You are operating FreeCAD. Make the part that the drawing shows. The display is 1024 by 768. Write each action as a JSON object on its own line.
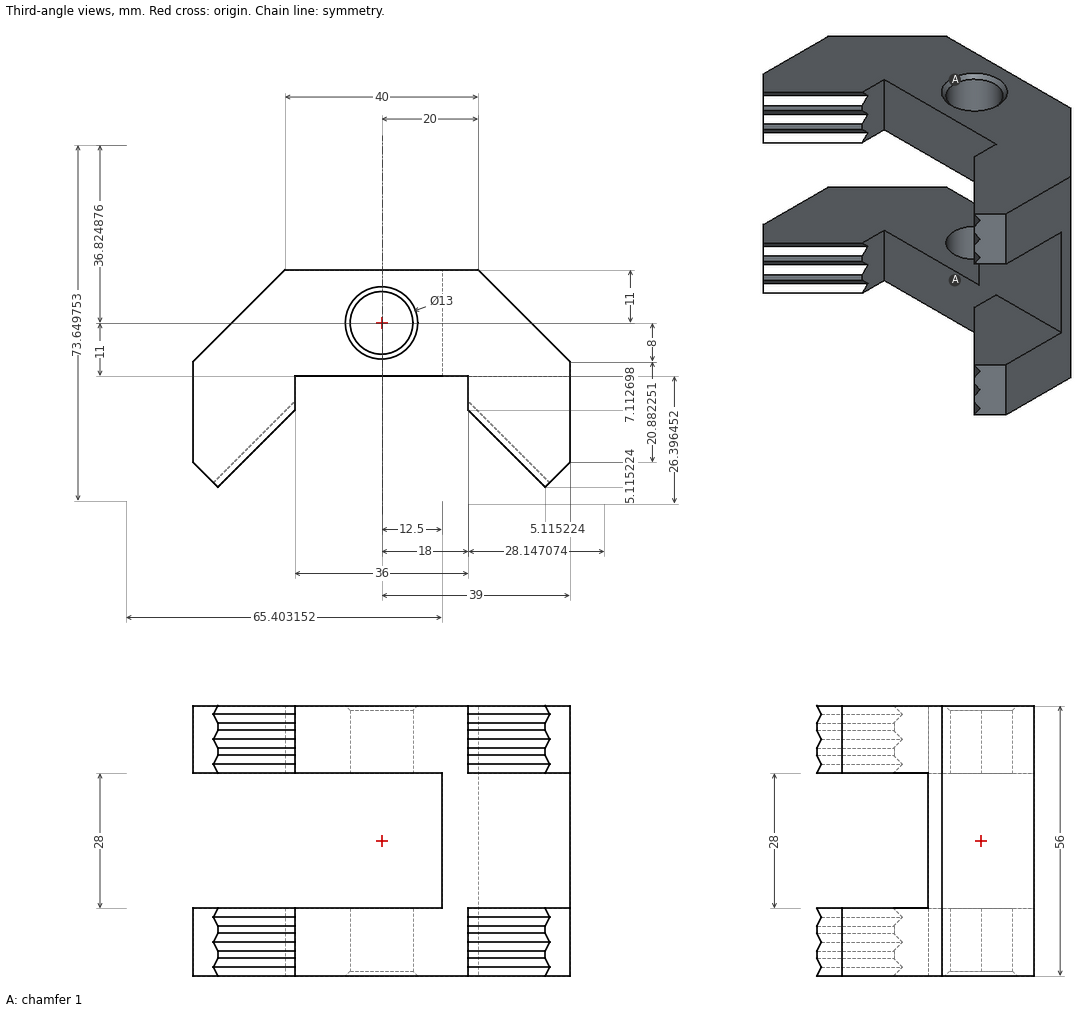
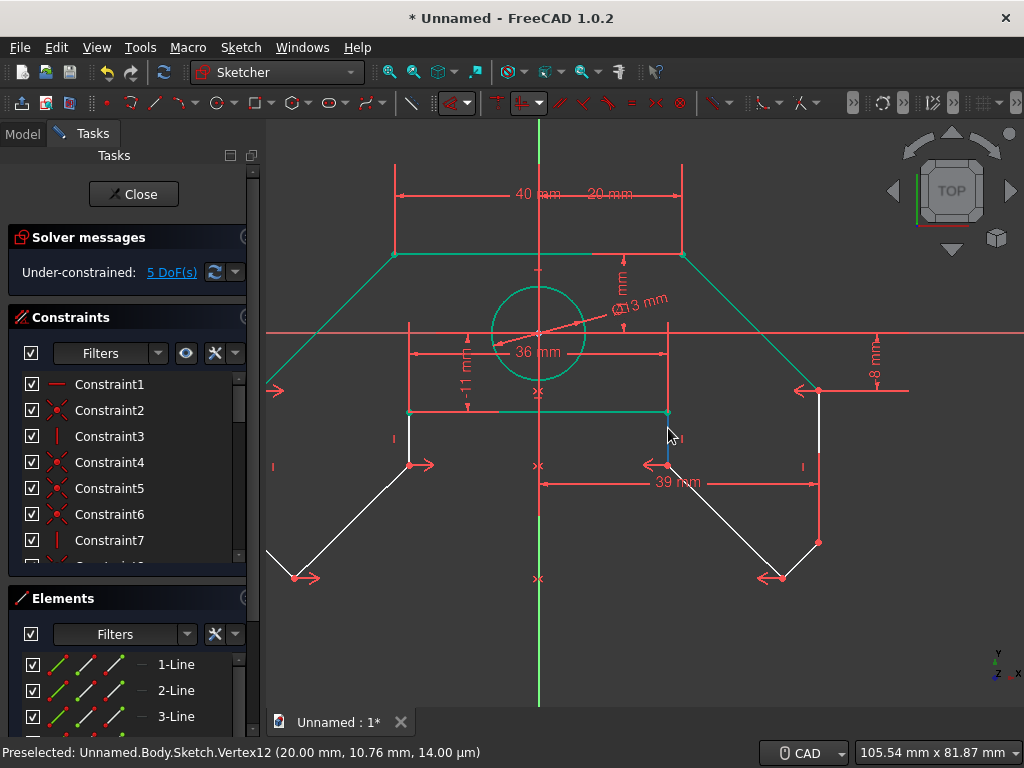
{"action": "left_click", "coordinate": [668, 428]}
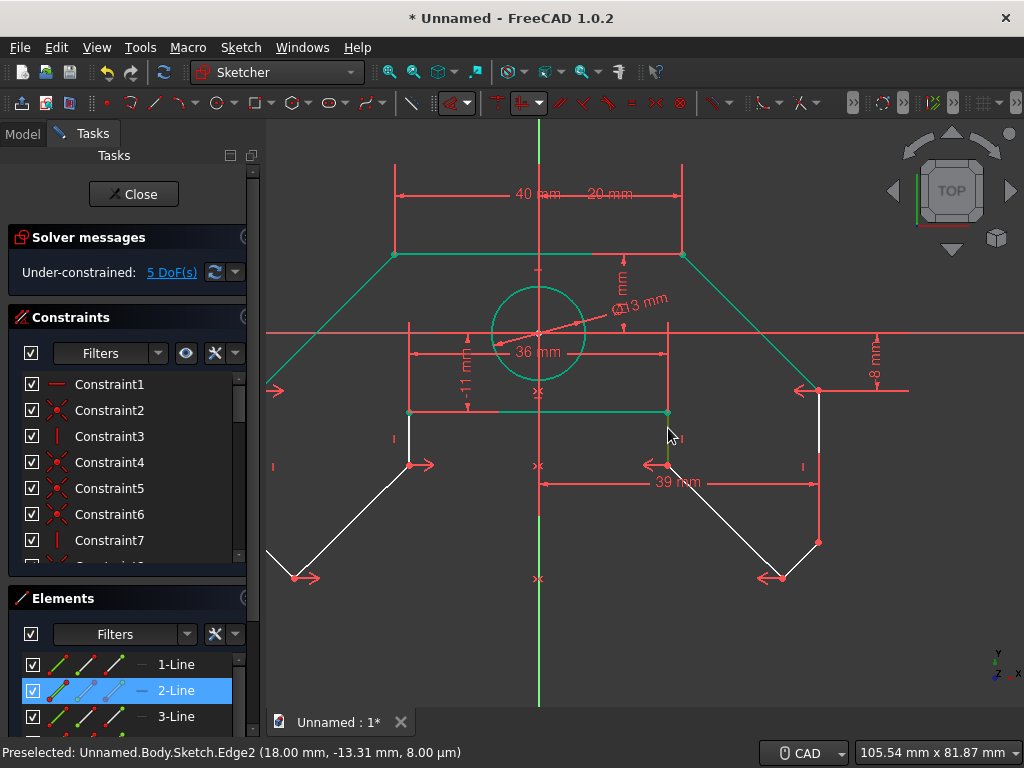
{"action": "key", "text": "i"}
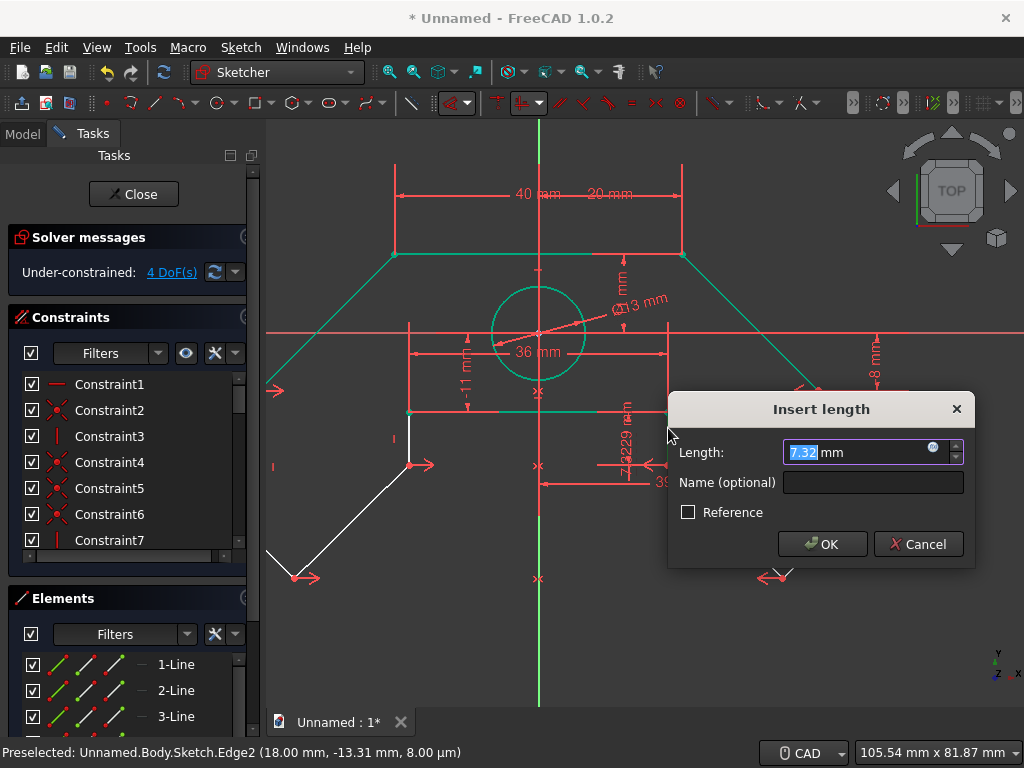
{"action": "type", "text": "7.112698"}
{"action": "key", "text": "Return"}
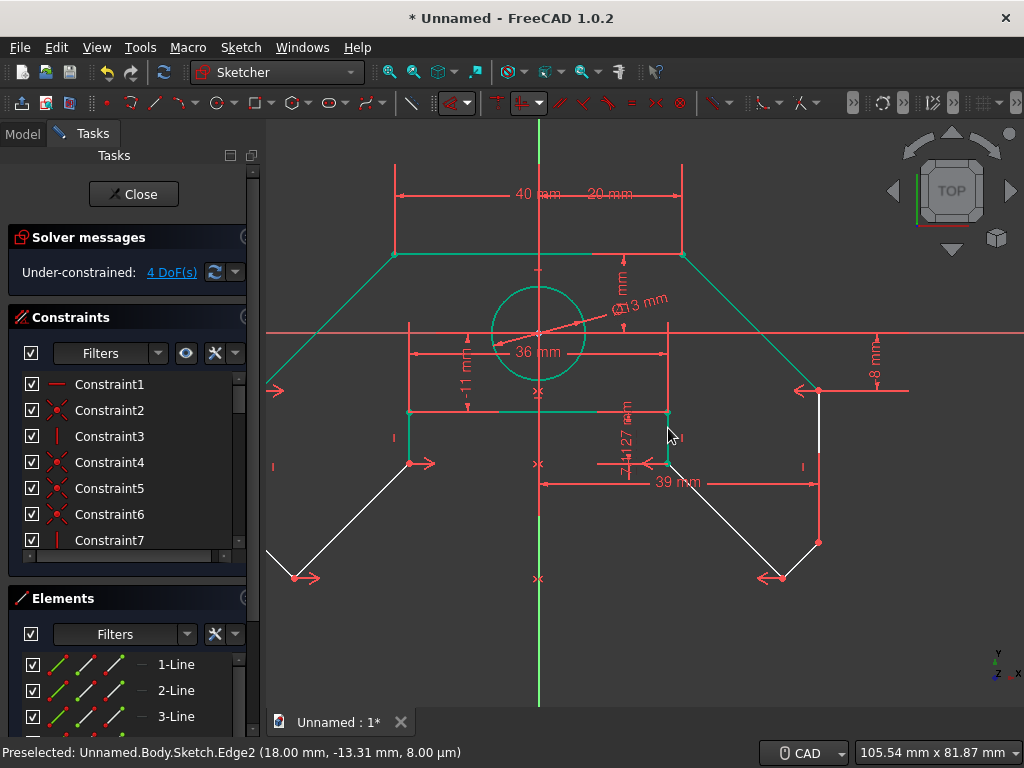
{"action": "left_click", "coordinate": [819, 497]}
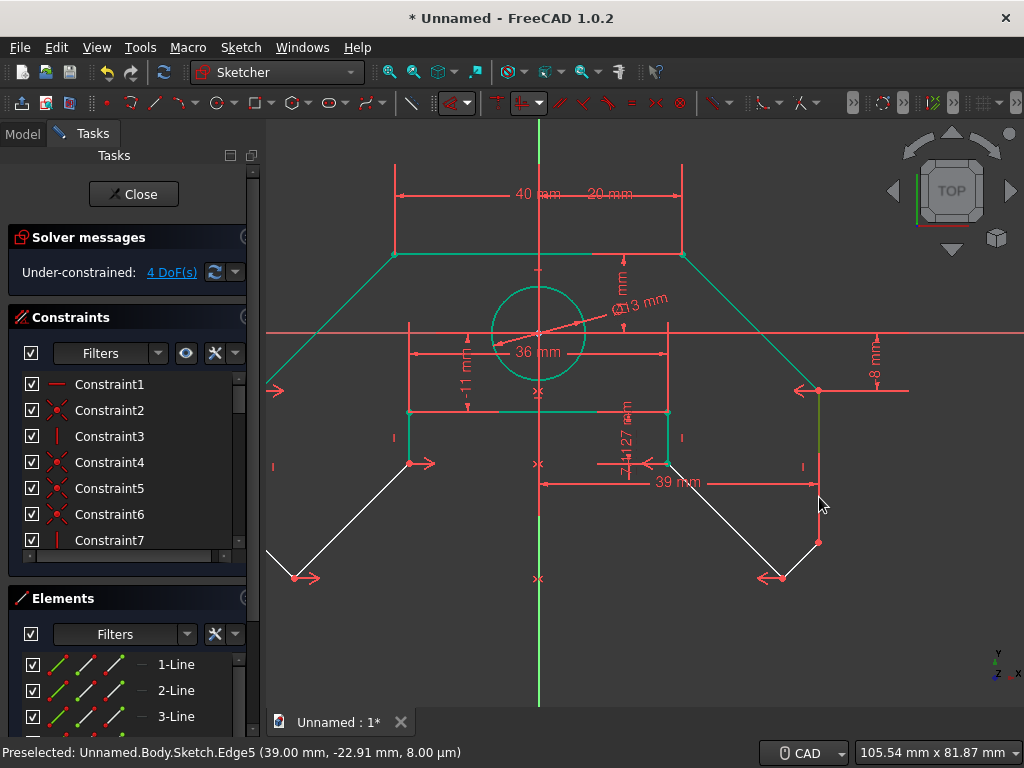
{"action": "key", "text": "i"}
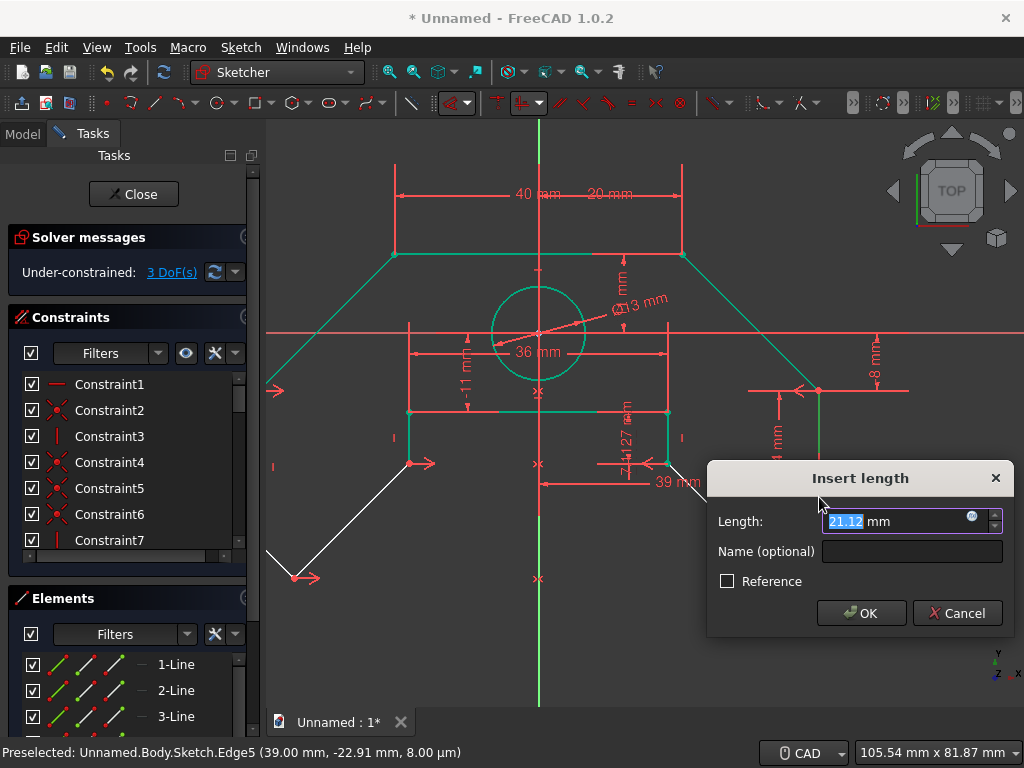
{"action": "type", "text": "20.882251"}
{"action": "key", "text": "Return"}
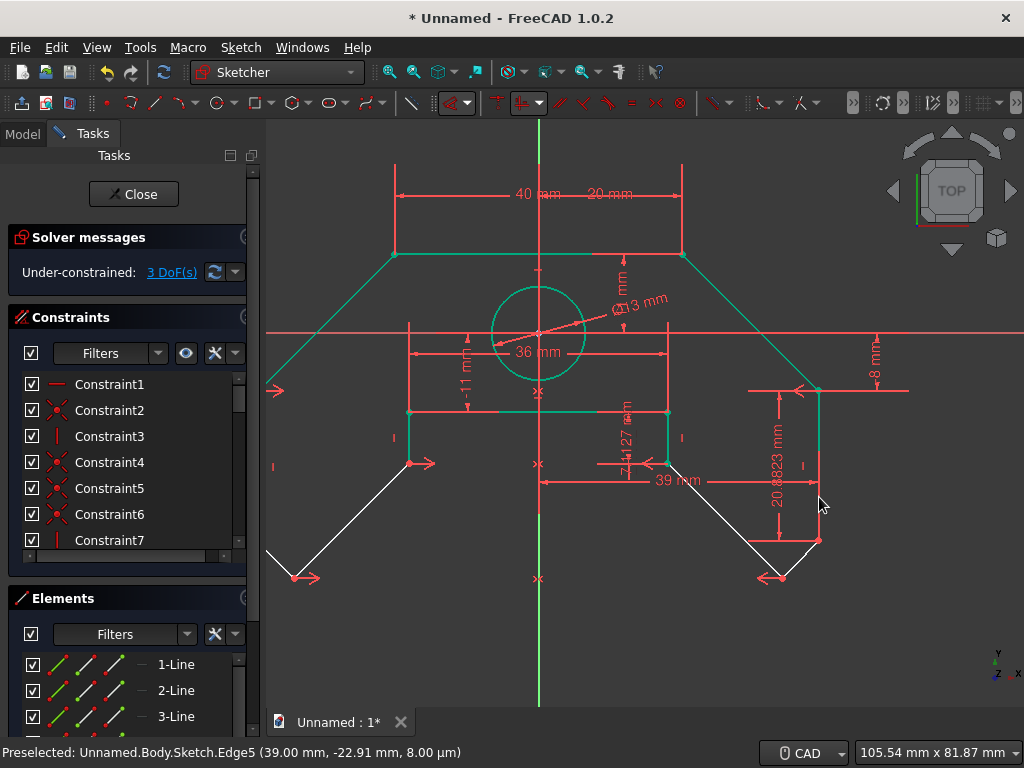
{"action": "scroll", "coordinate": [654, 407], "scroll_direction": "down", "scroll_amount": 2}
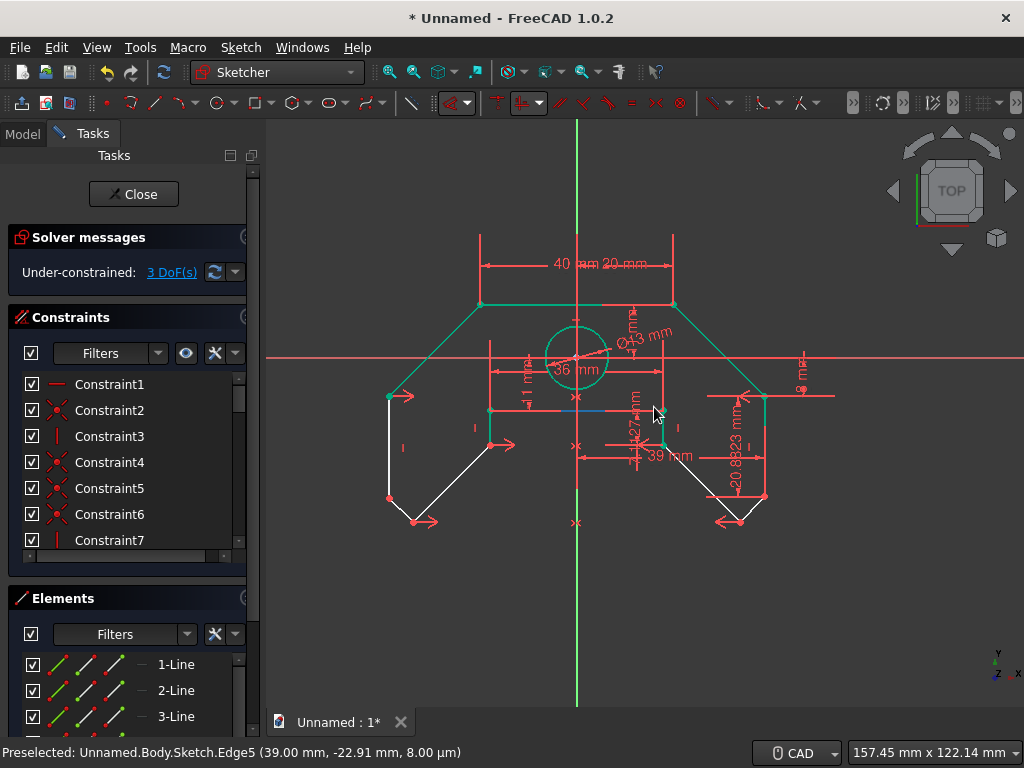
{"action": "left_click", "coordinate": [389, 427]}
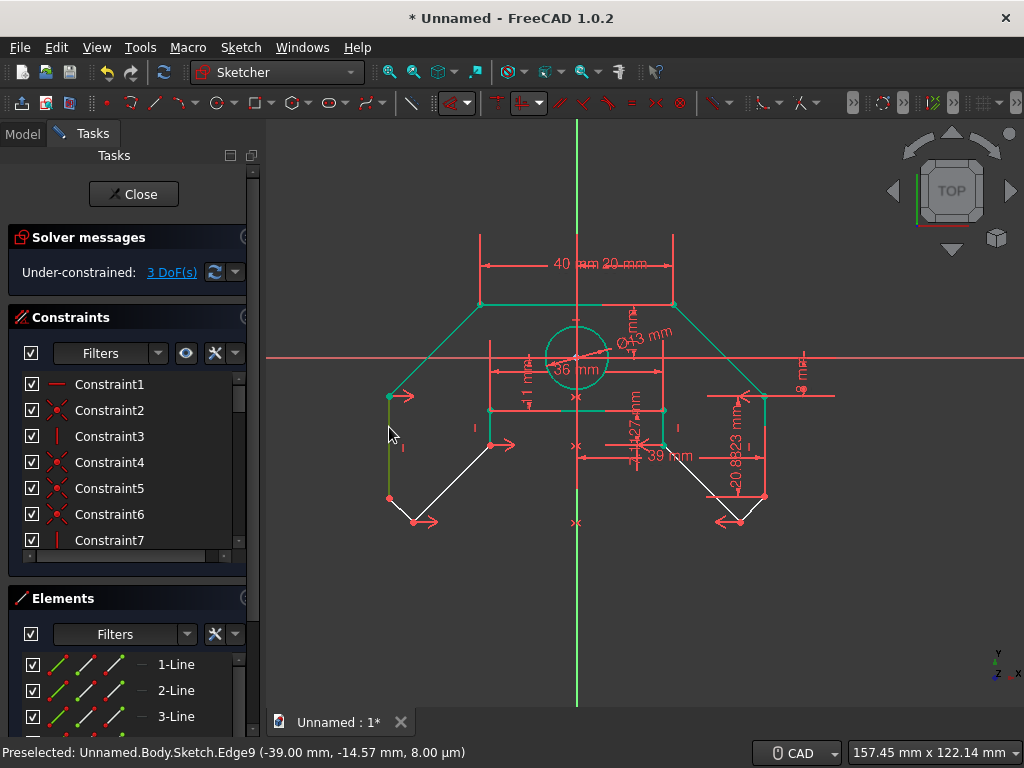
{"action": "key", "text": "i"}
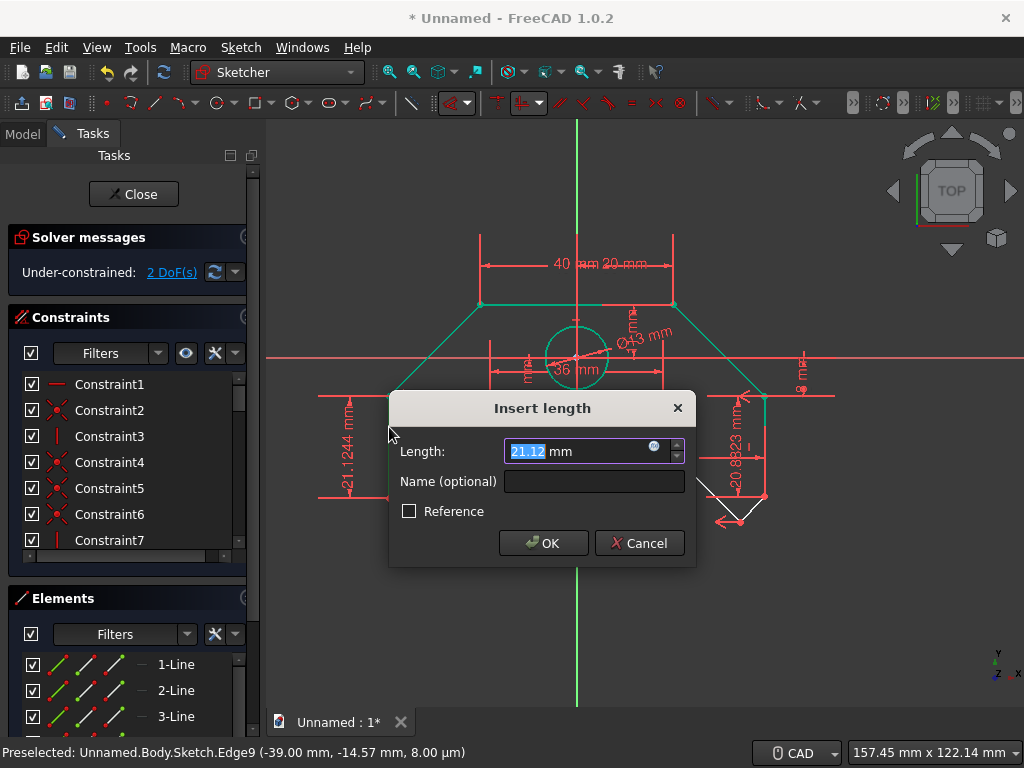
{"action": "type", "text": "20.882251"}
{"action": "key", "text": "Return"}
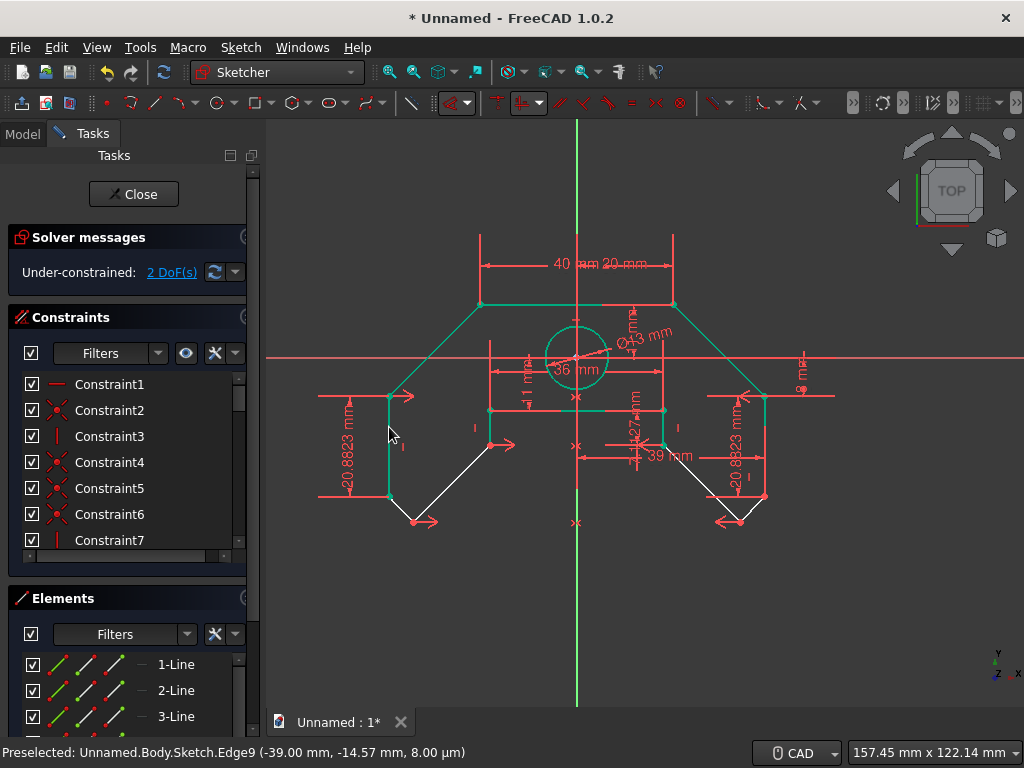
{"action": "scroll", "coordinate": [748, 515], "scroll_direction": "up", "scroll_amount": 3}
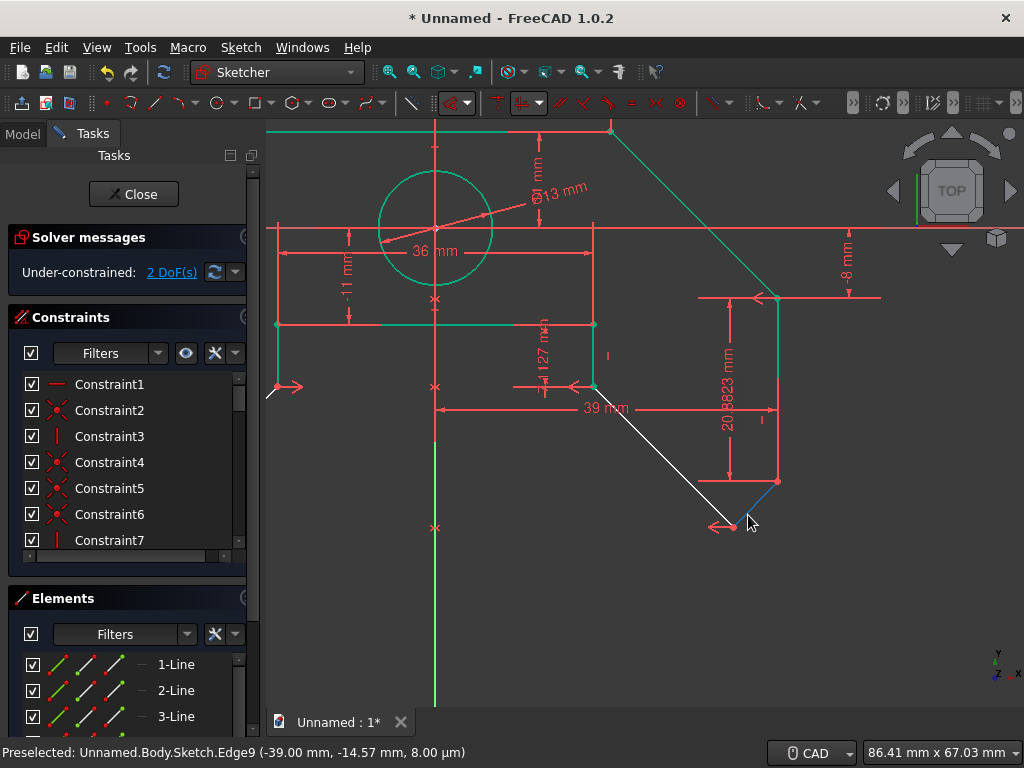
{"action": "left_click", "coordinate": [747, 514]}